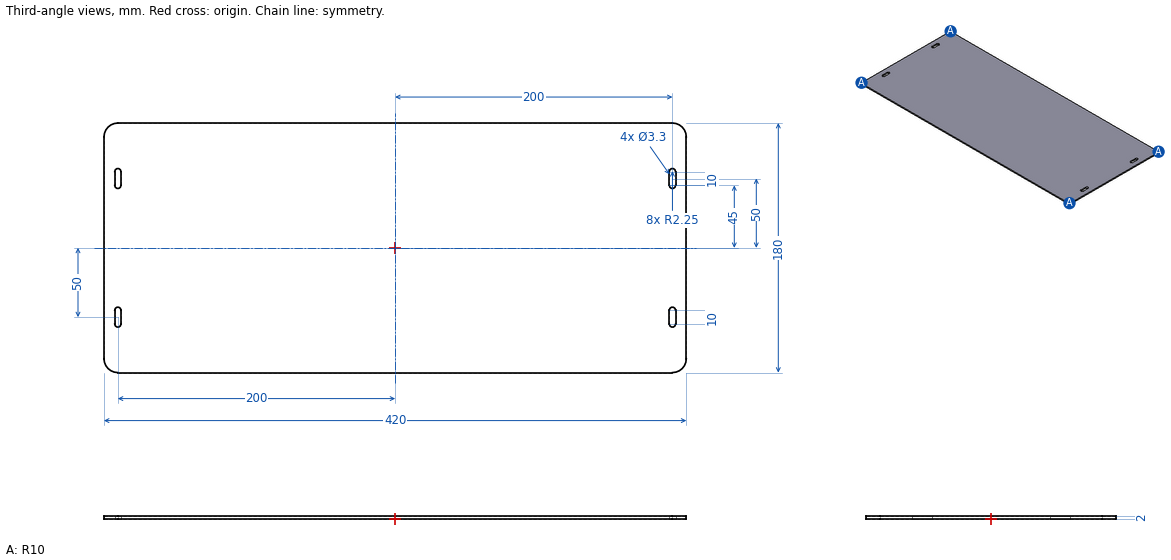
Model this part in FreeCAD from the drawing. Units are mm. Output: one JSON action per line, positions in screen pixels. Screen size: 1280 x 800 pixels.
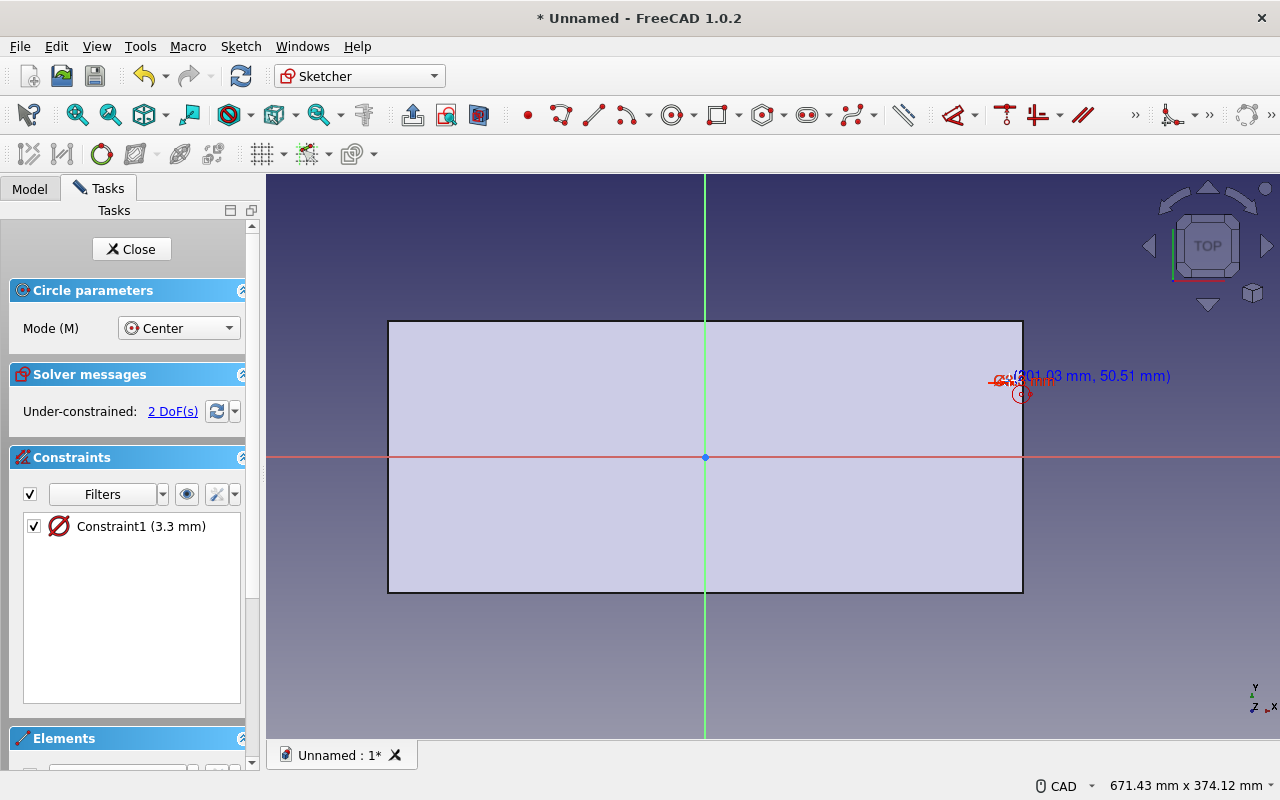
{"action": "scroll", "coordinate": [403, 533], "scroll_direction": "up", "scroll_amount": 12}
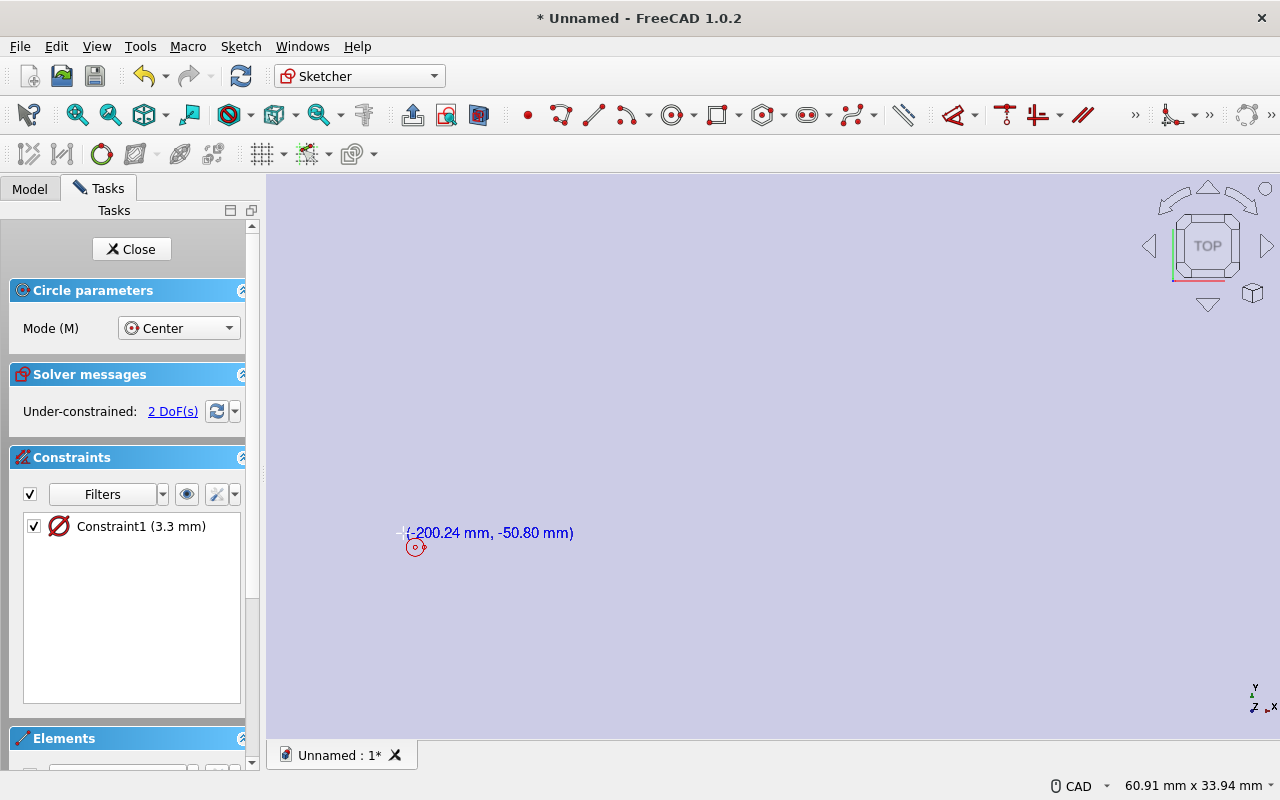
{"action": "scroll", "coordinate": [402, 533], "scroll_direction": "down", "scroll_amount": 12}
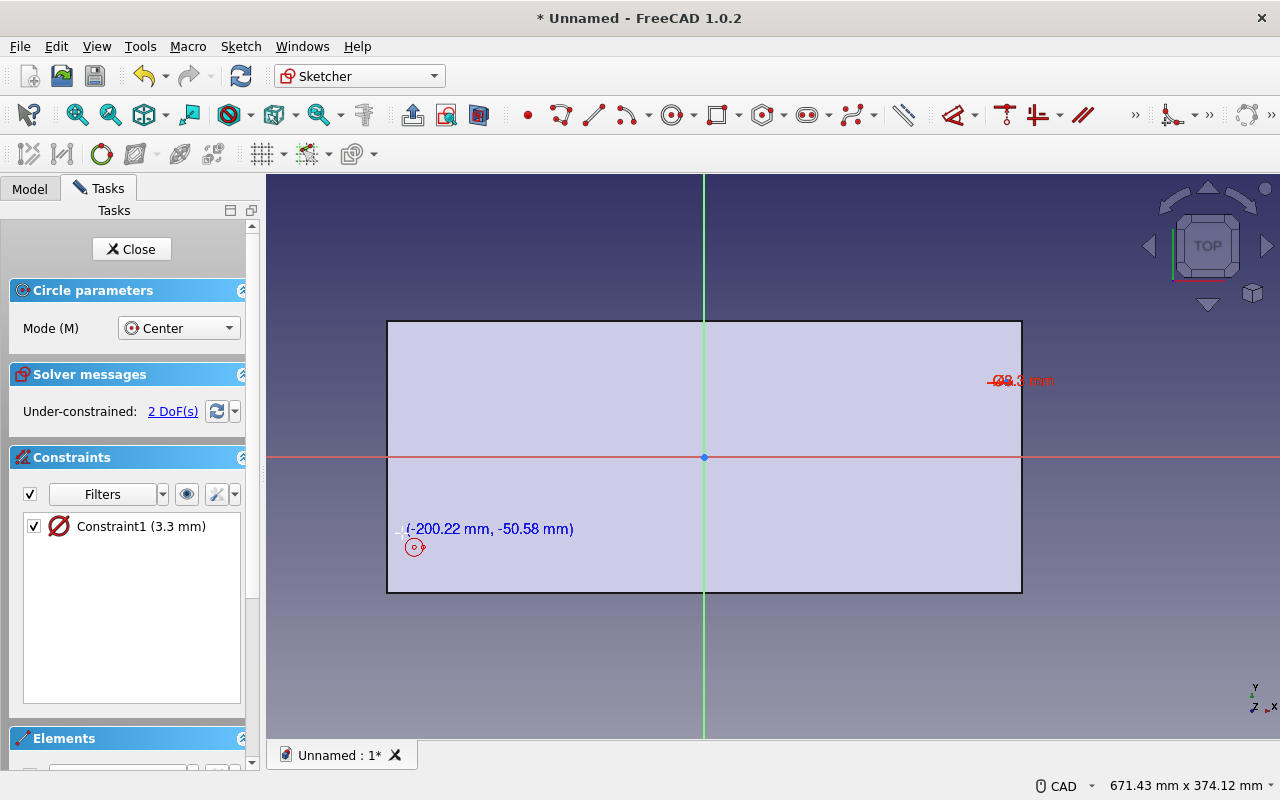
{"action": "left_click", "coordinate": [402, 533]}
{"action": "mouse_move", "coordinate": [404, 531]}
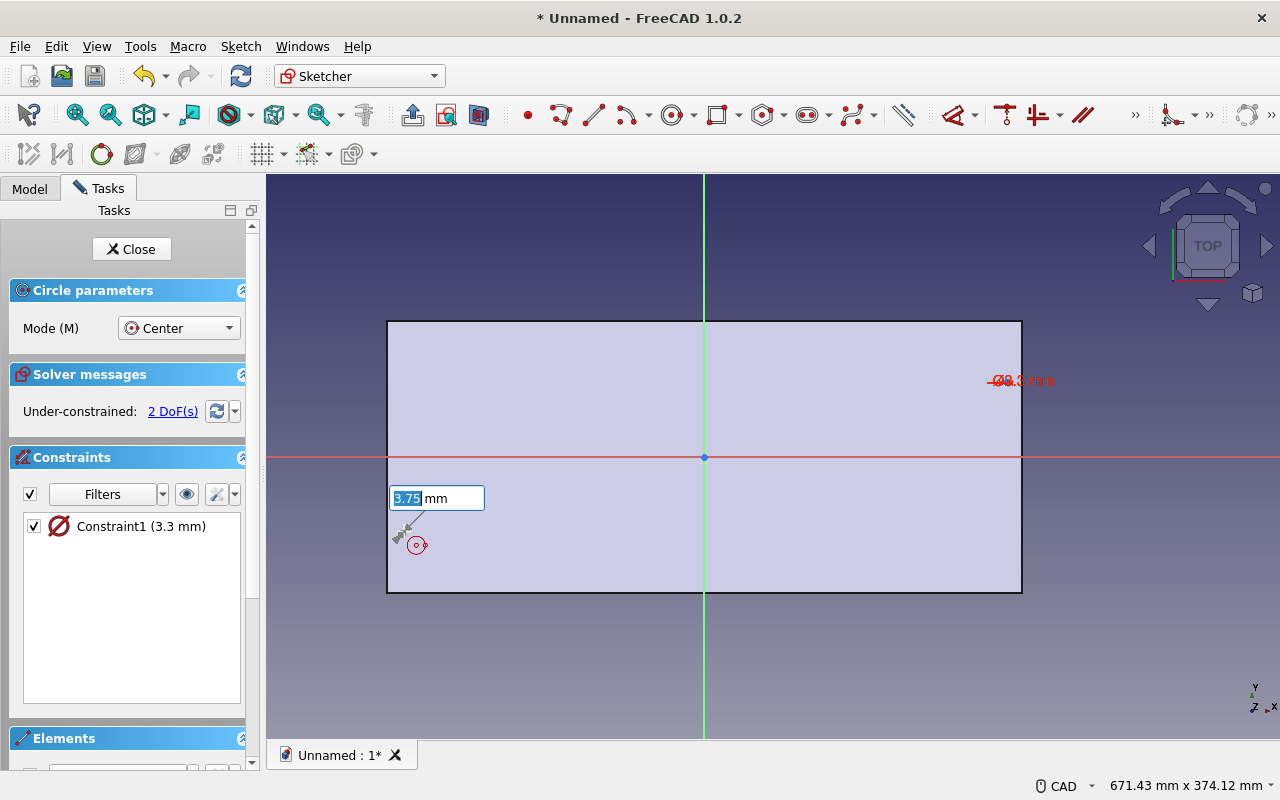
{"action": "type", "text": "3.3"}
{"action": "key", "text": "Return"}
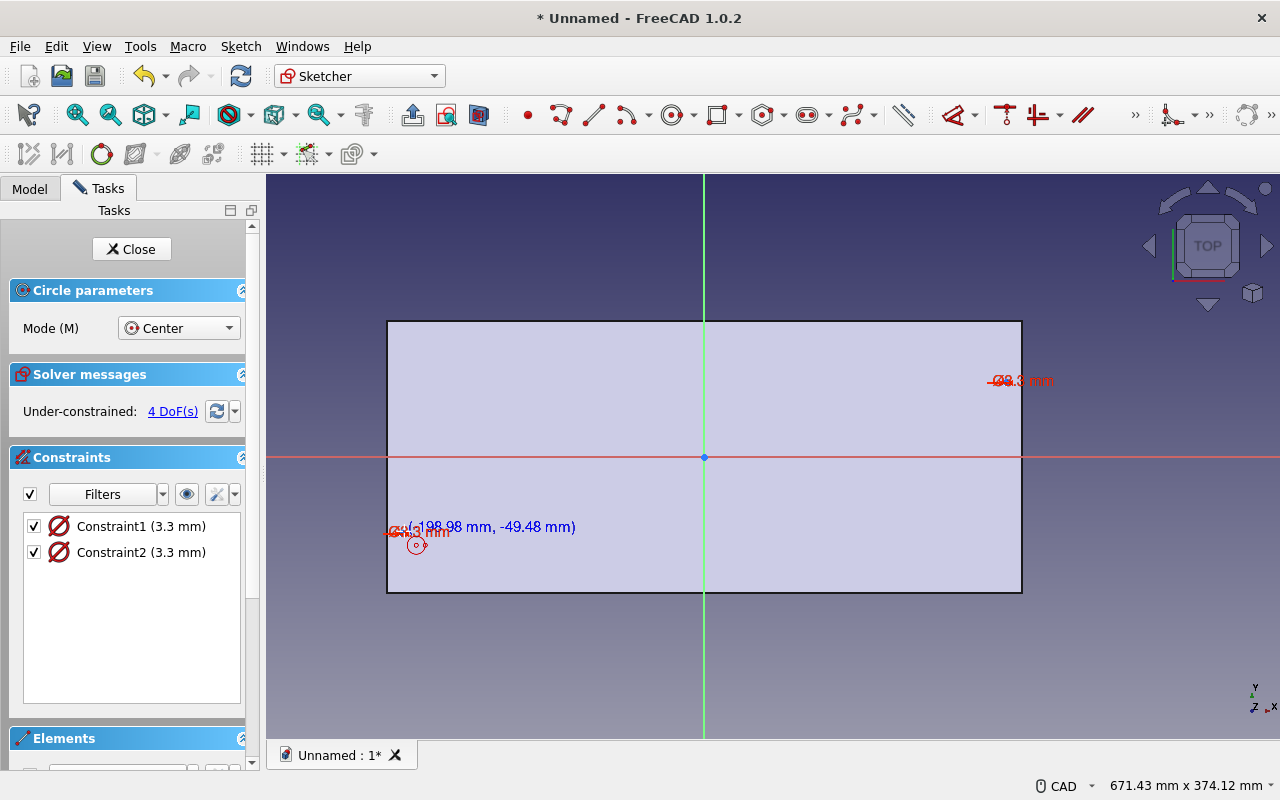
{"action": "scroll", "coordinate": [402, 382], "scroll_direction": "up", "scroll_amount": 12}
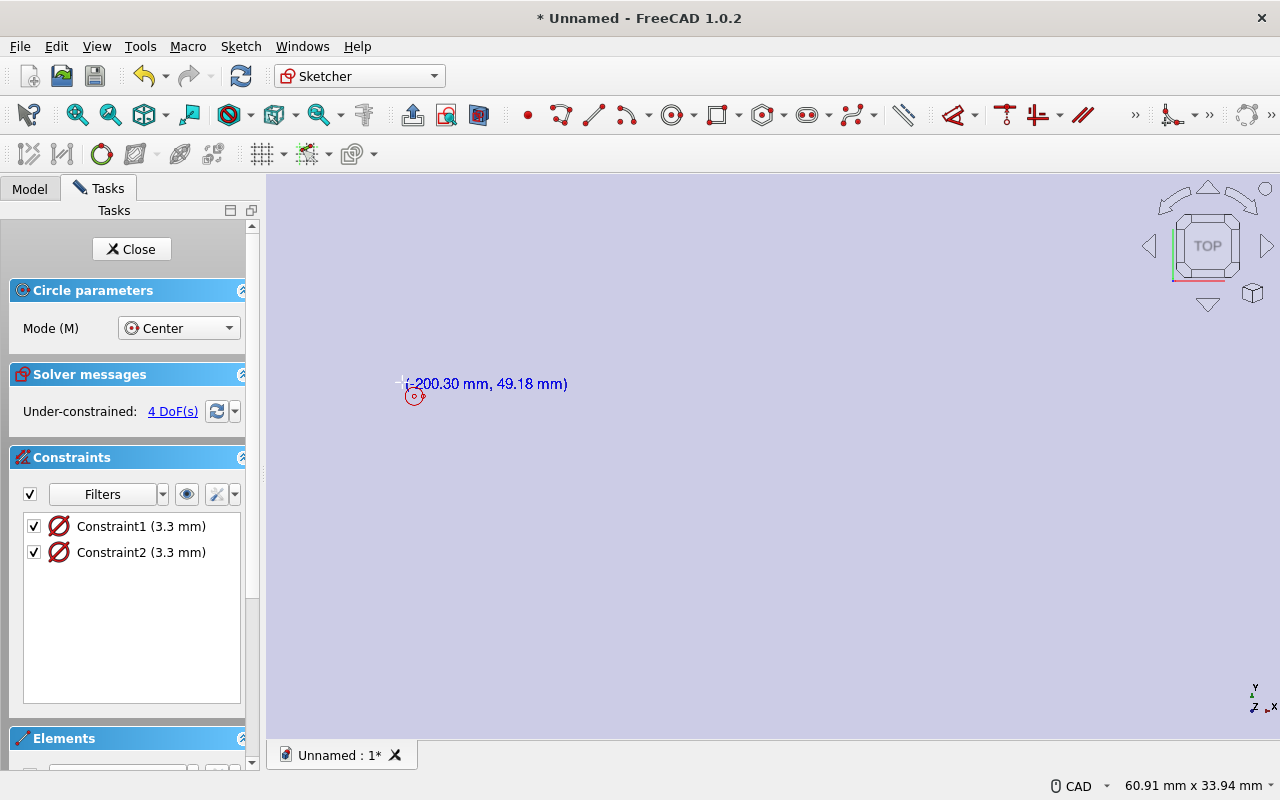
{"action": "scroll", "coordinate": [402, 382], "scroll_direction": "down", "scroll_amount": 12}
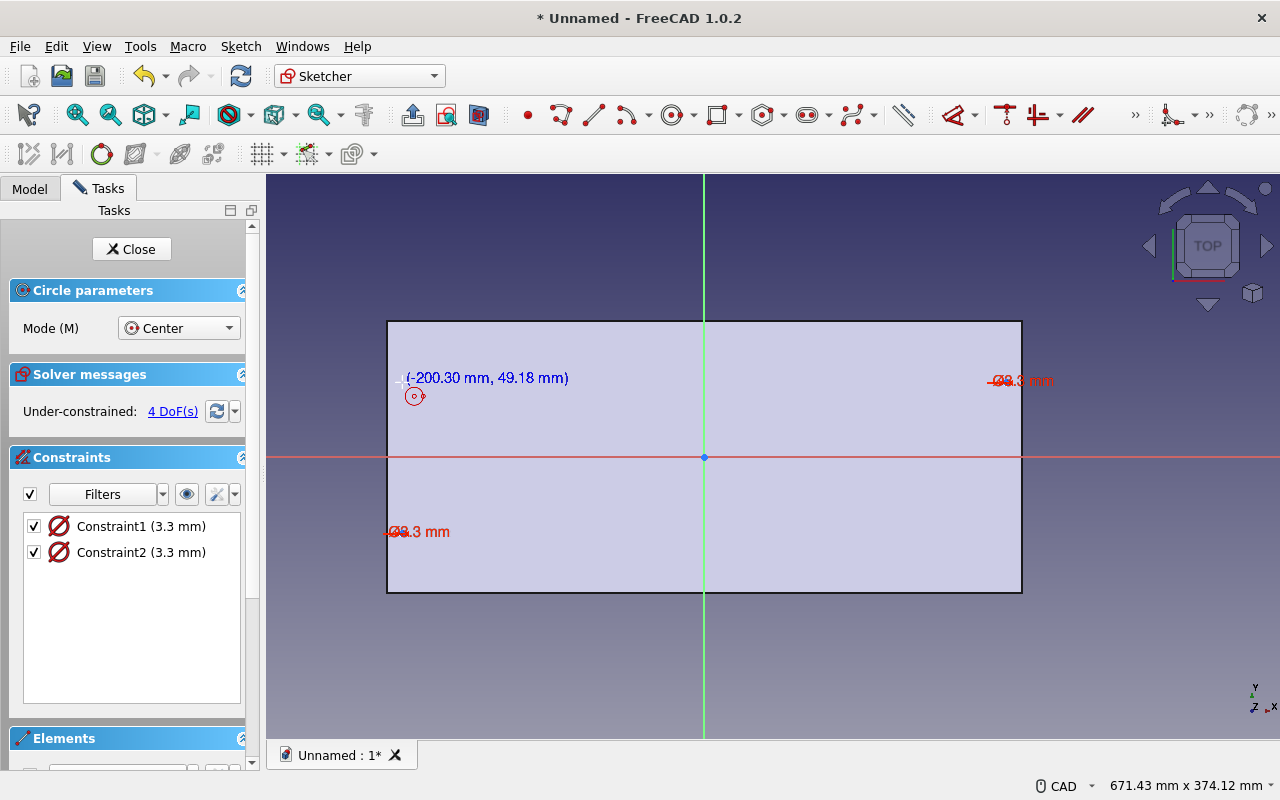
{"action": "left_click", "coordinate": [402, 382]}
{"action": "mouse_move", "coordinate": [404, 380]}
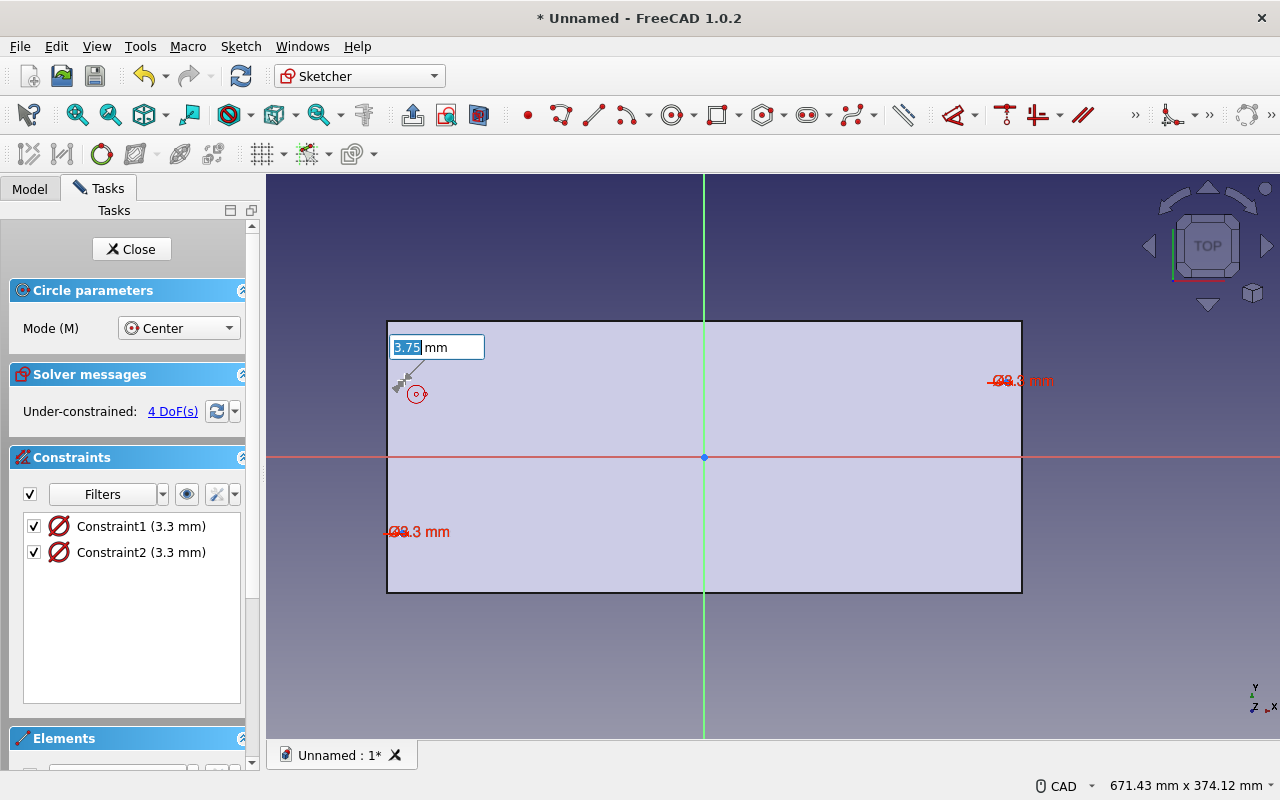
{"action": "type", "text": "3.3"}
{"action": "key", "text": "Return"}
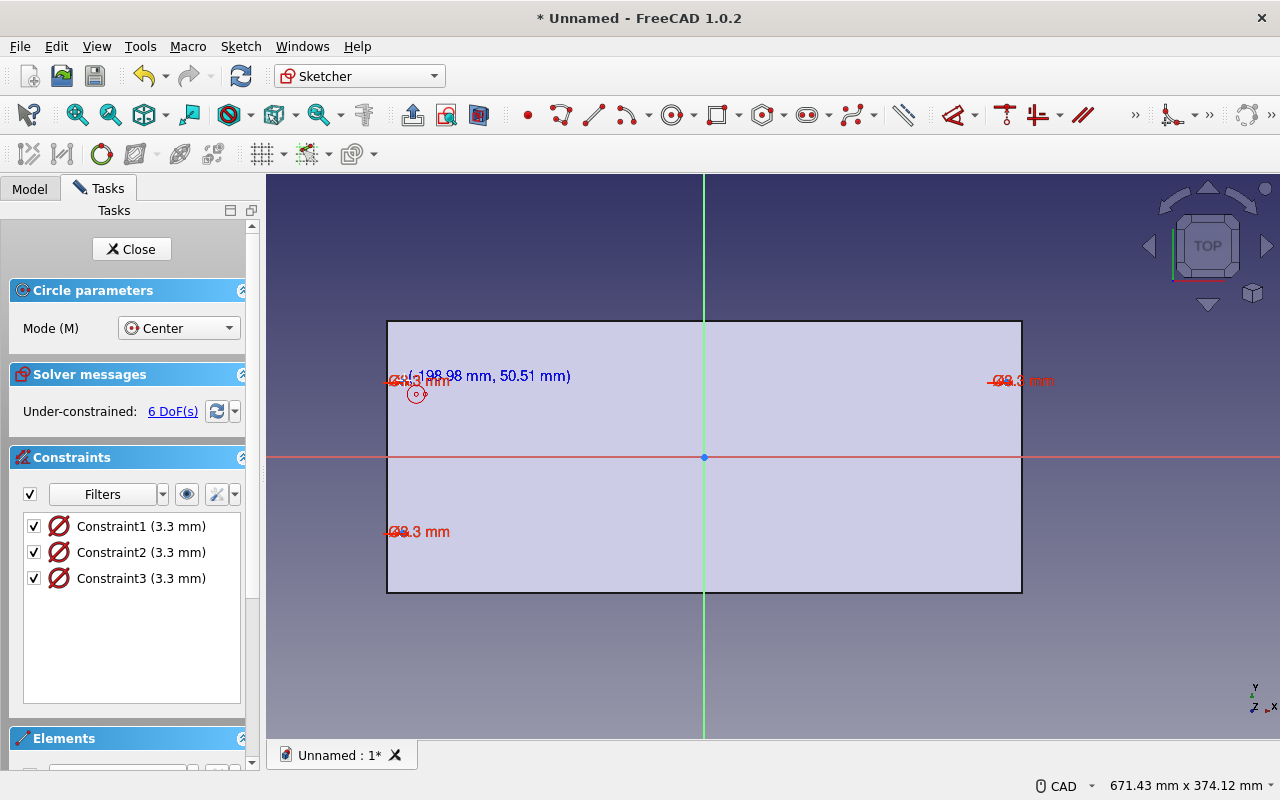
{"action": "scroll", "coordinate": [1007, 533], "scroll_direction": "up", "scroll_amount": 12}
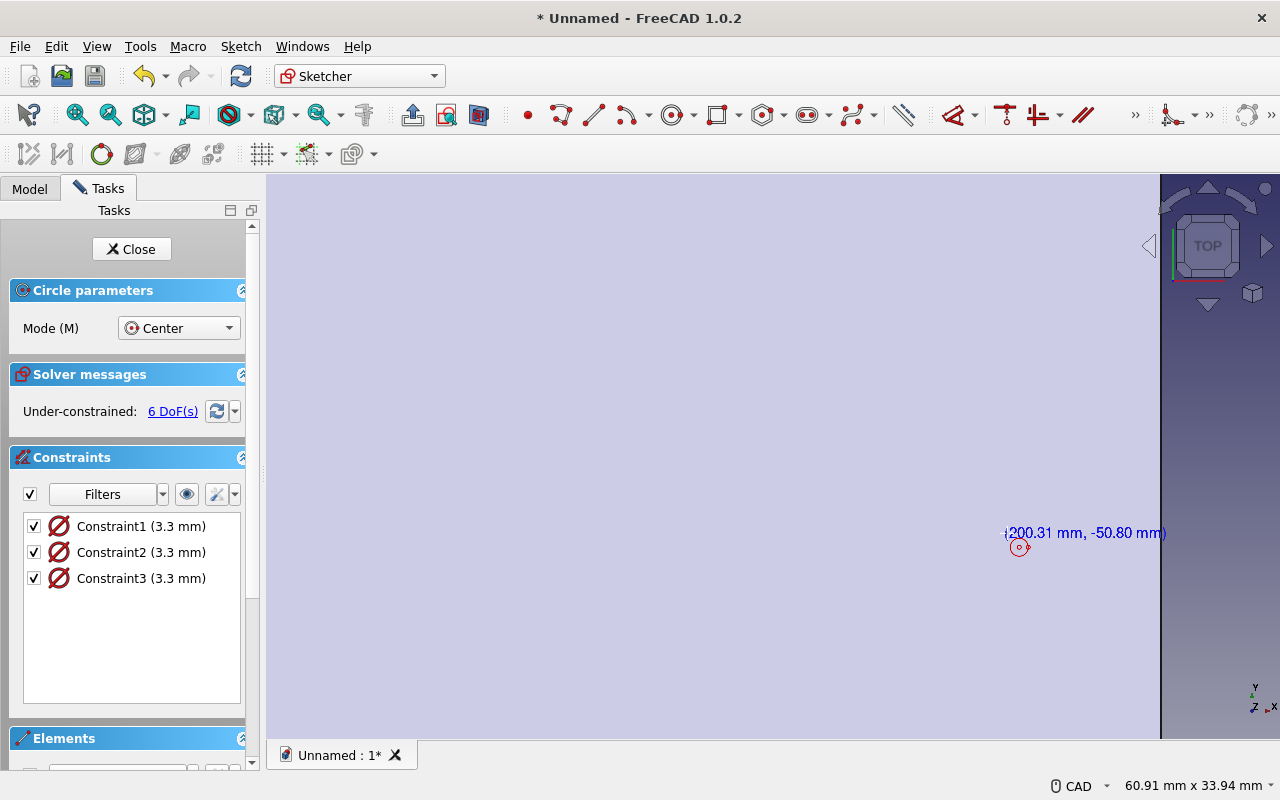
{"action": "scroll", "coordinate": [1008, 533], "scroll_direction": "down", "scroll_amount": 12}